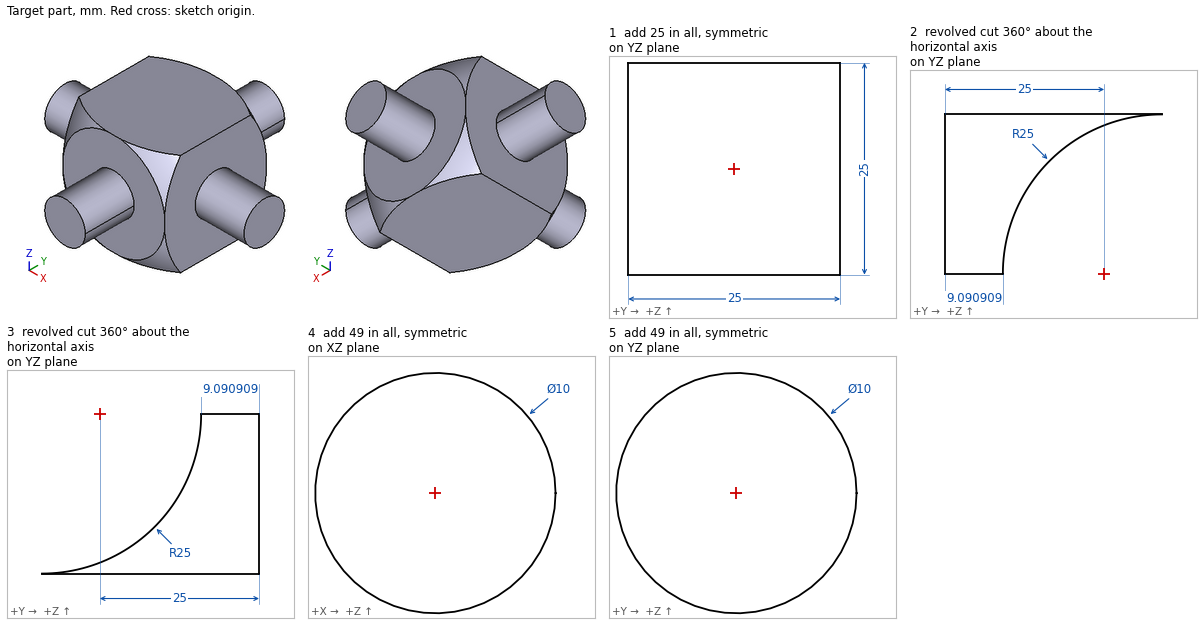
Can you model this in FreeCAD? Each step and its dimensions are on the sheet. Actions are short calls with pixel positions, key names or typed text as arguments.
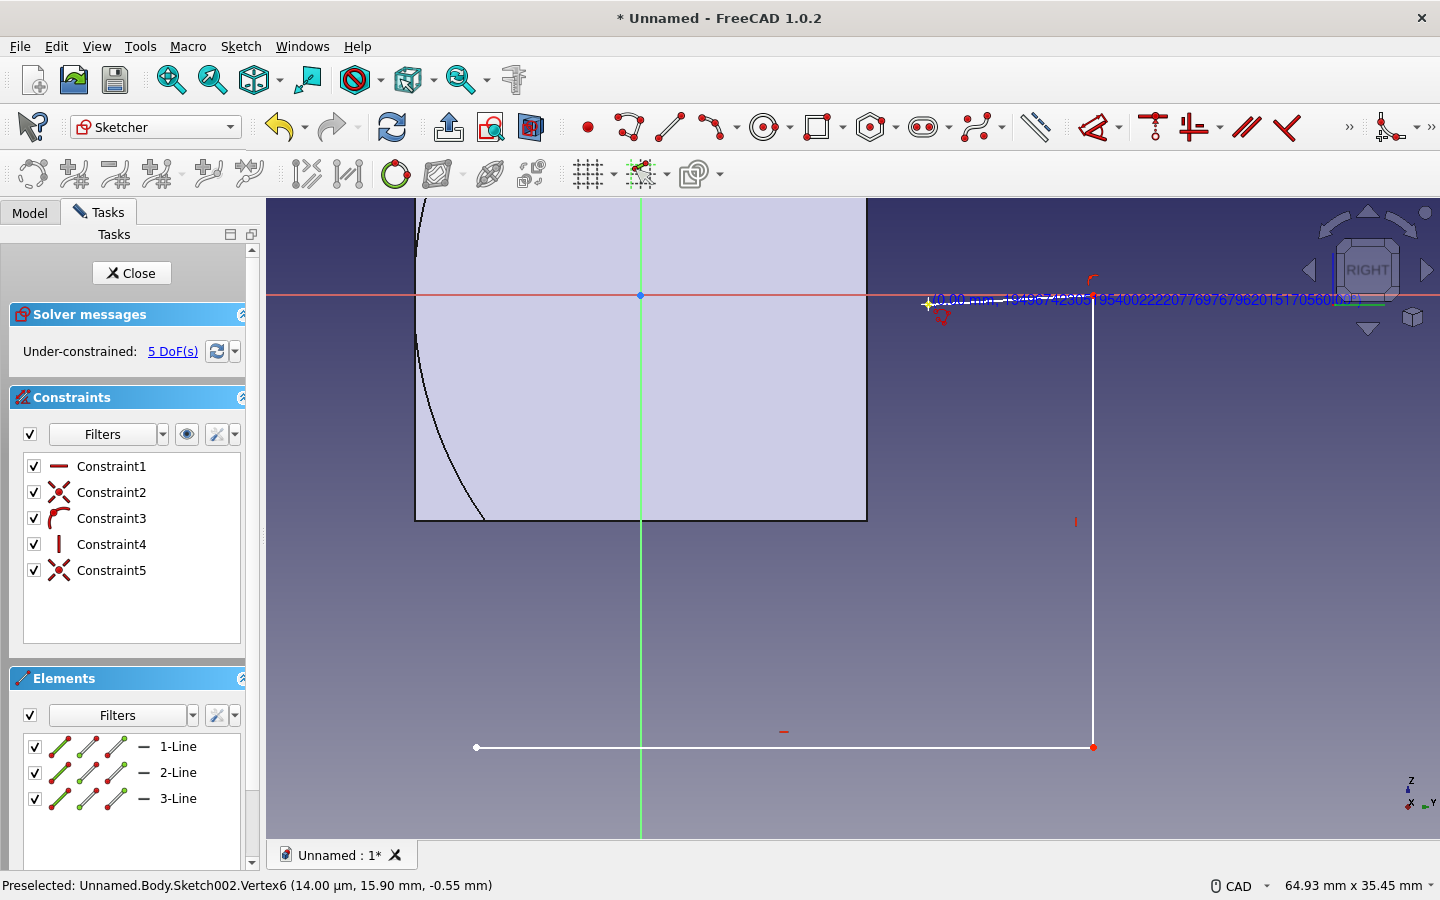
key(g)
key(3)
key(a)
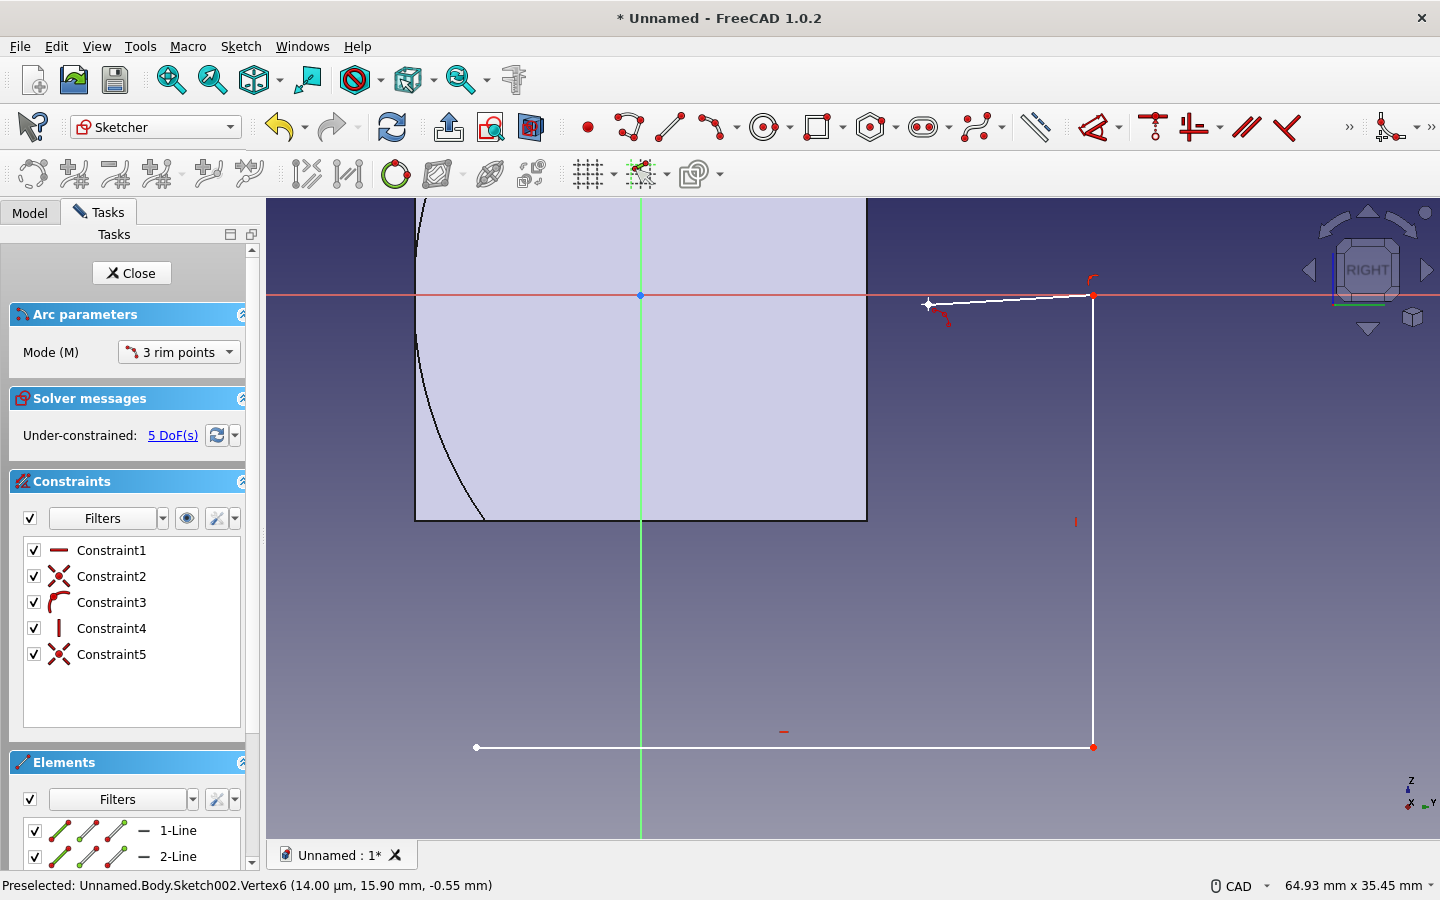
click(928, 305)
click(476, 748)
click(796, 615)
key(Escape)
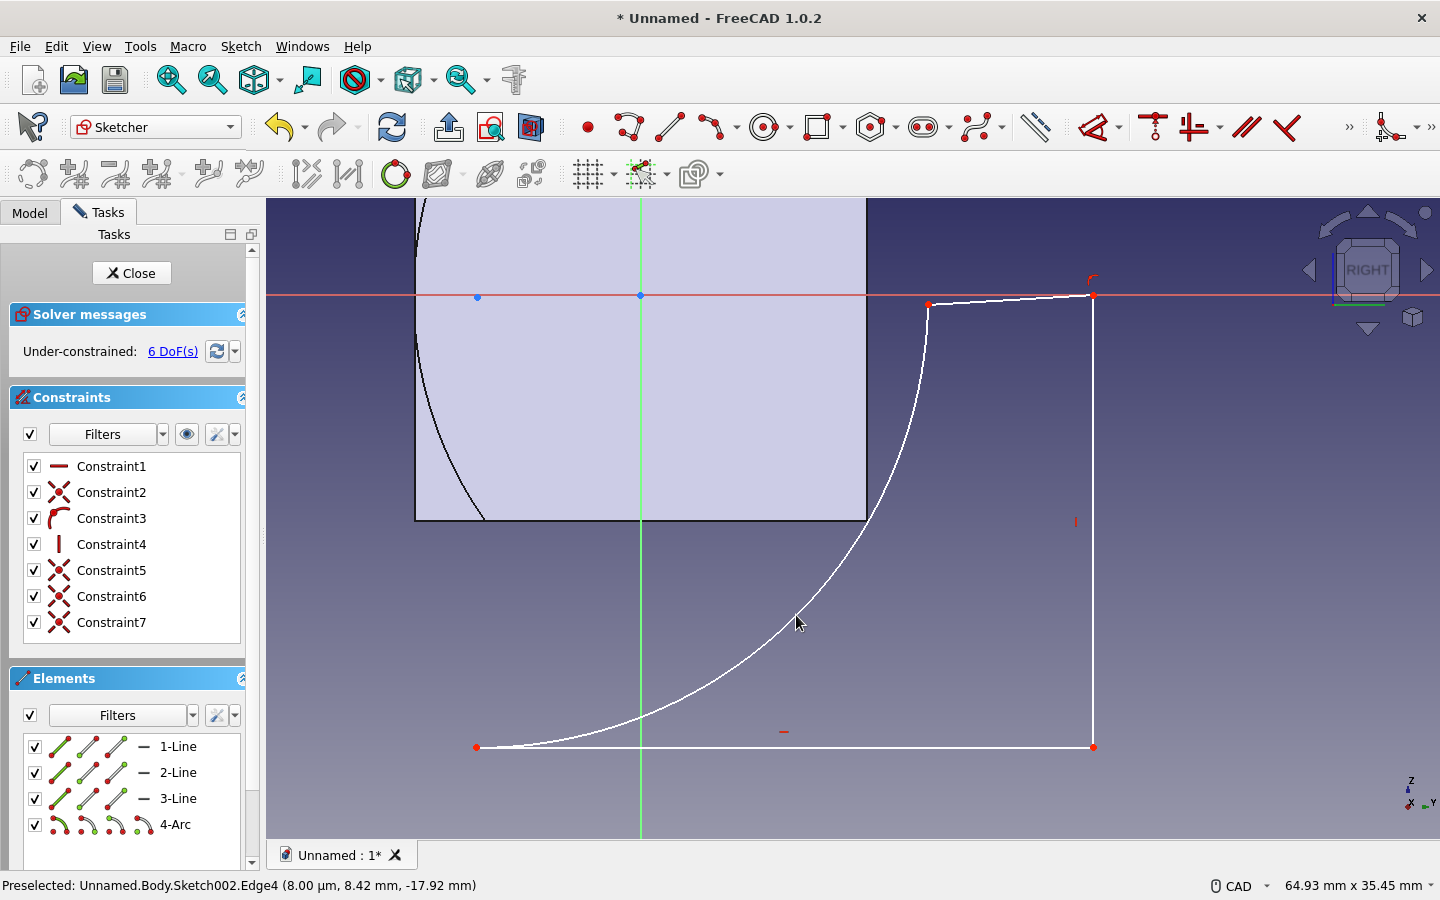
click(661, 748)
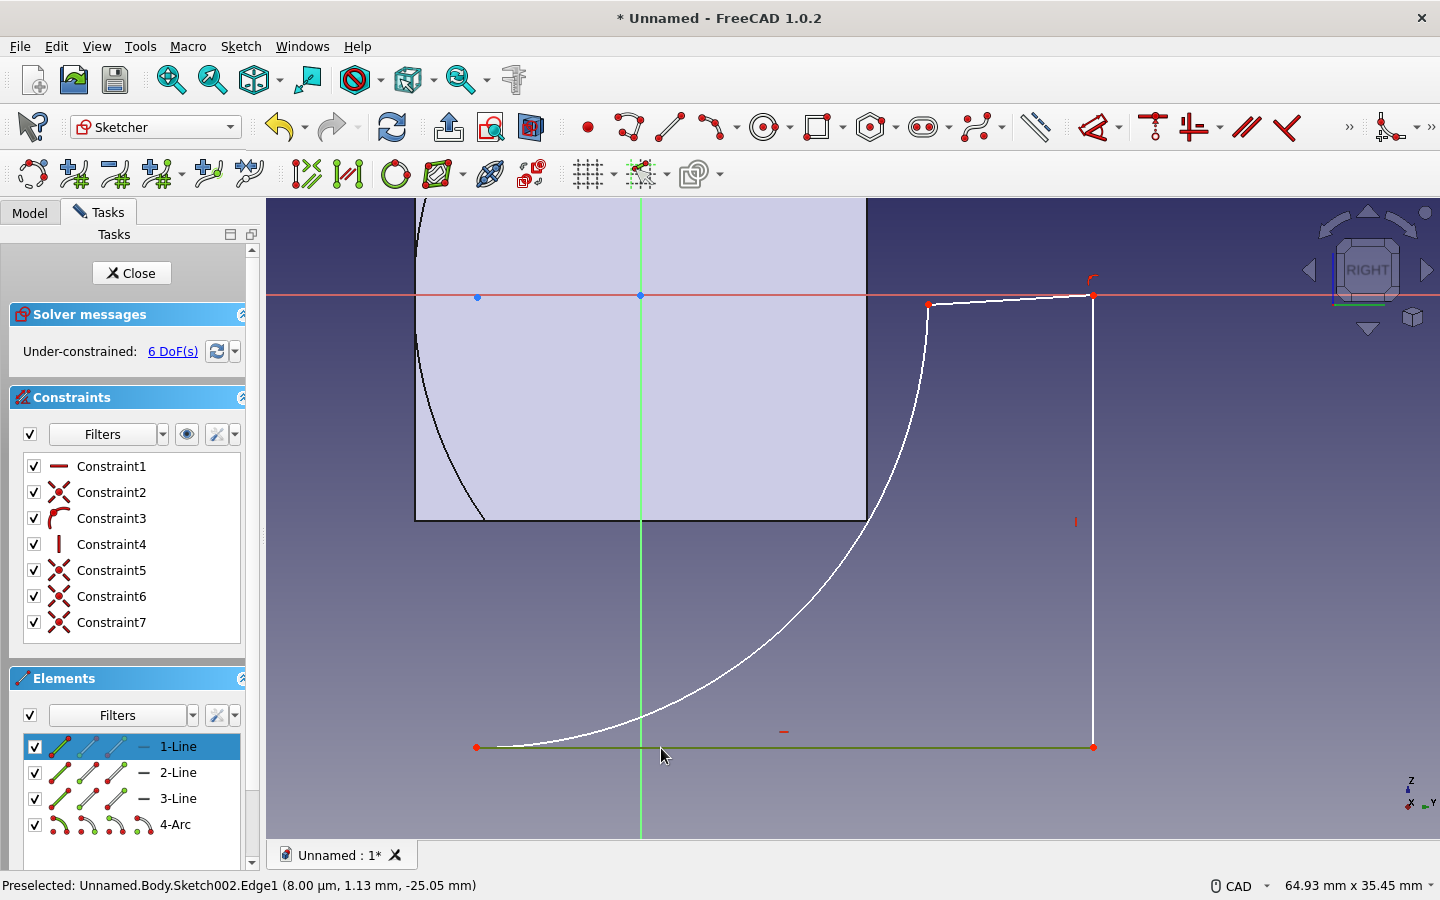
click(679, 700)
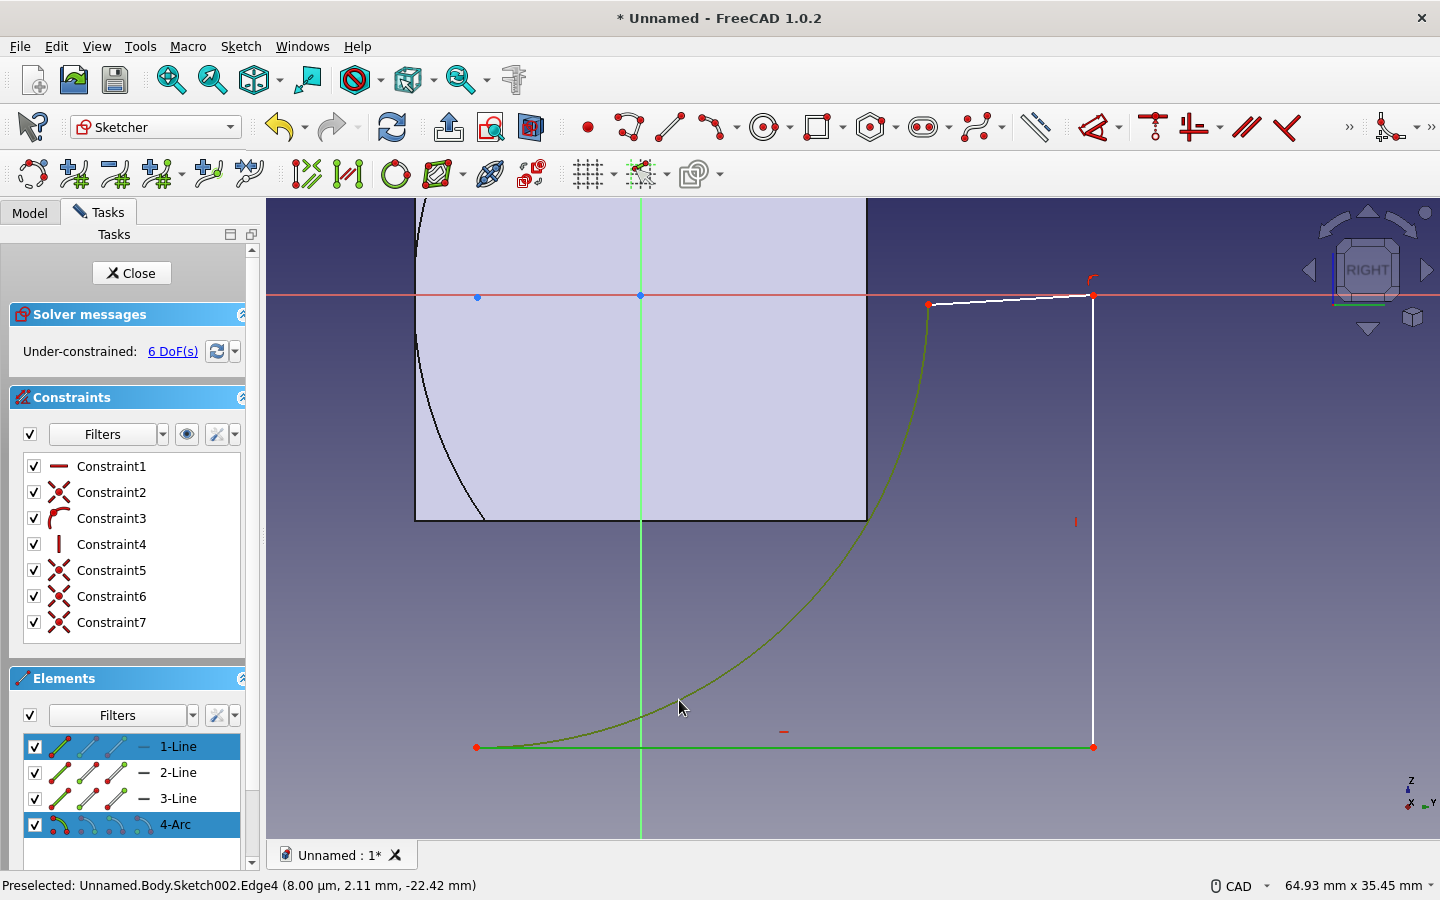
key(t)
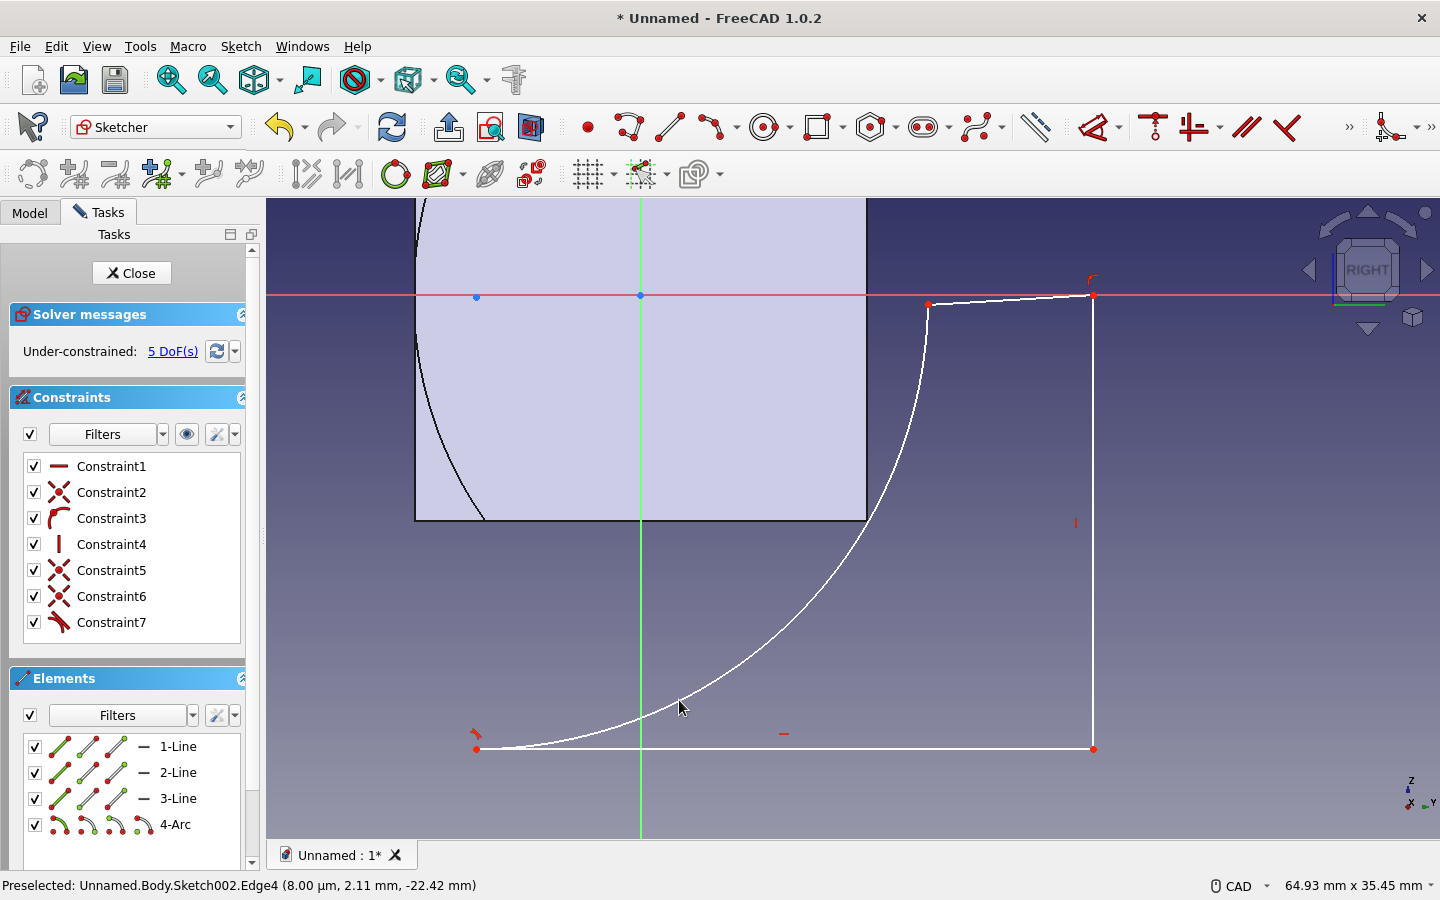
click(1044, 298)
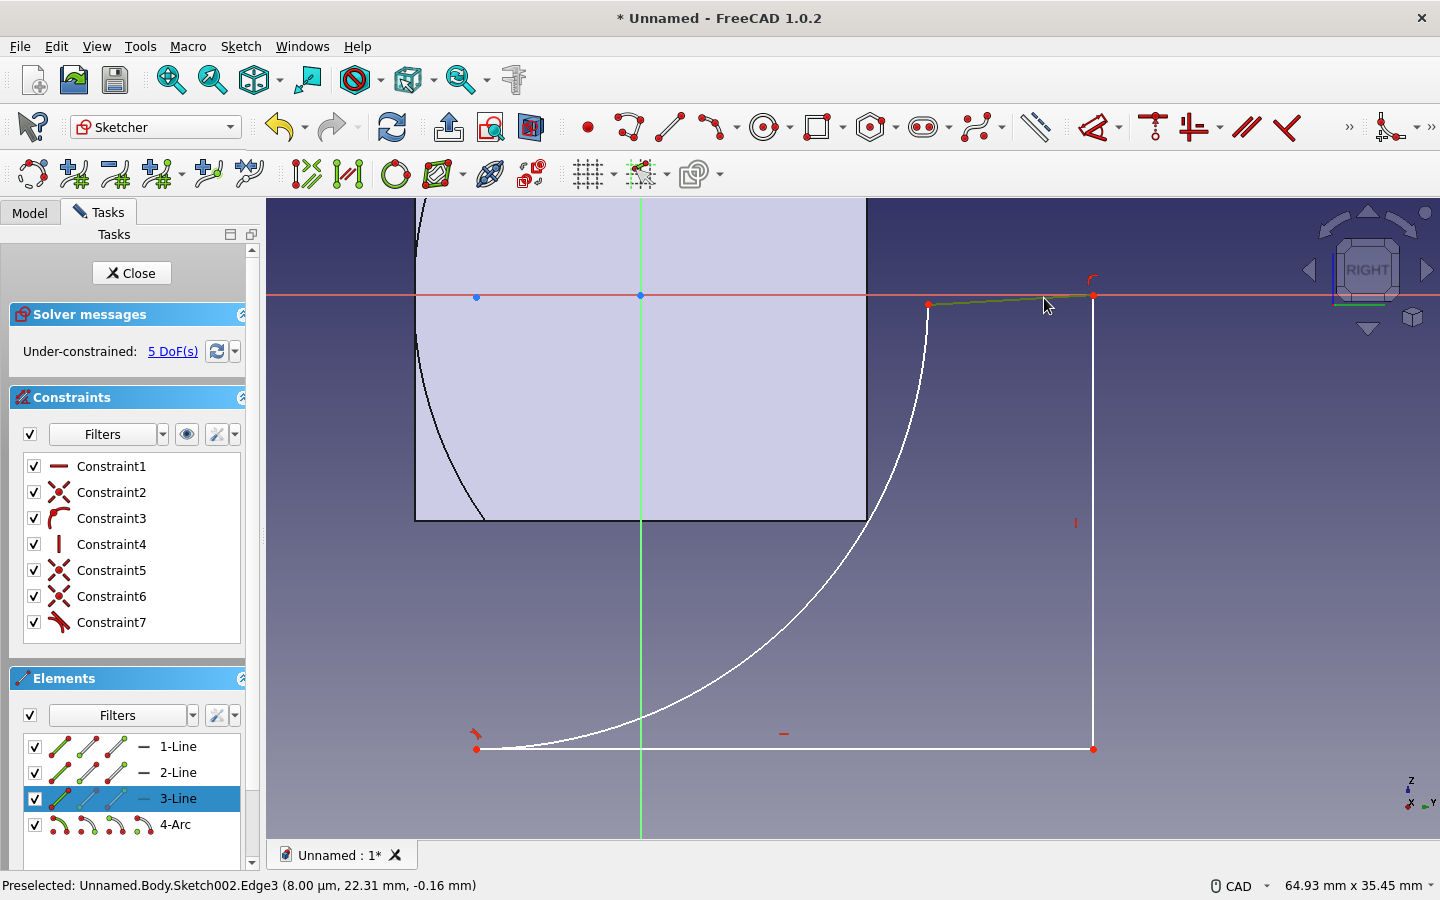
click(1220, 128)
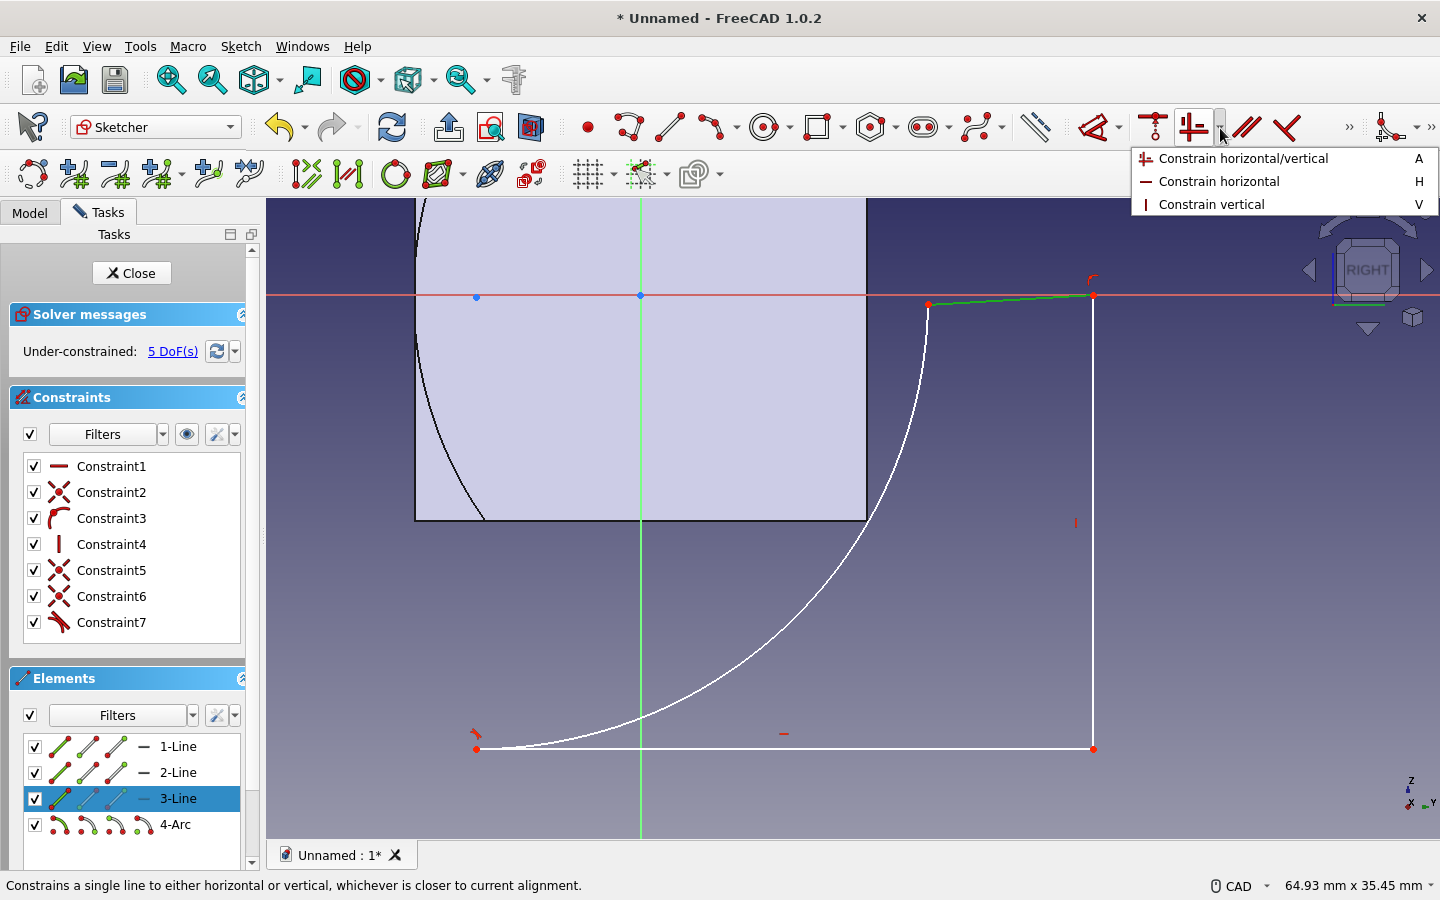
click(1285, 182)